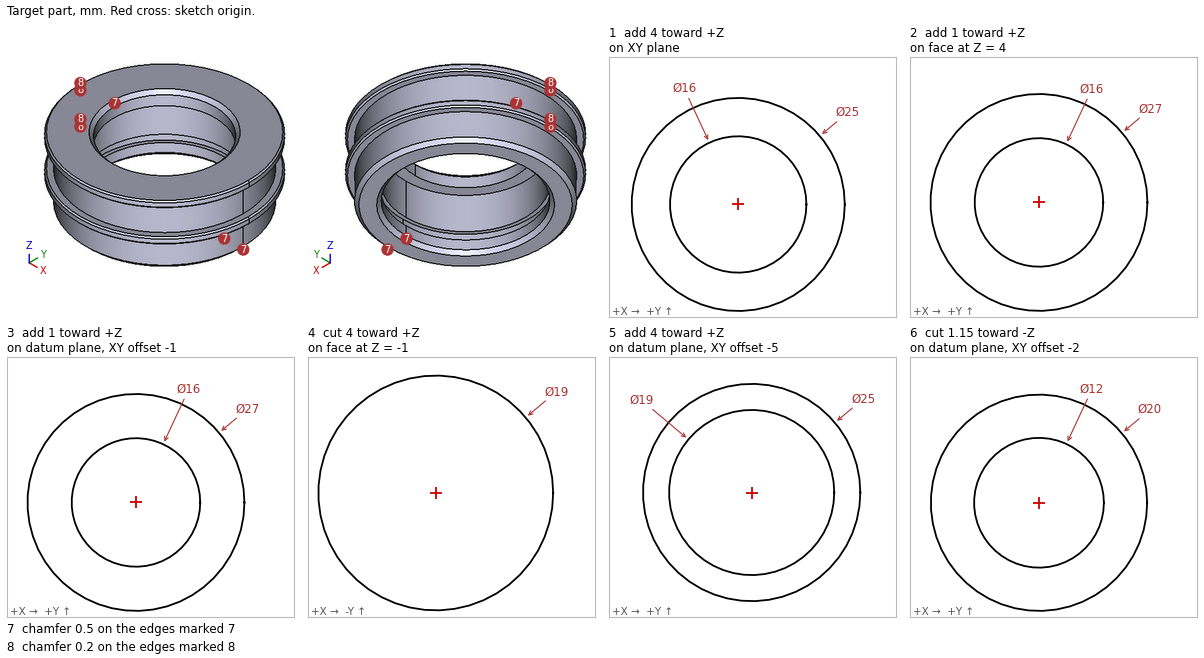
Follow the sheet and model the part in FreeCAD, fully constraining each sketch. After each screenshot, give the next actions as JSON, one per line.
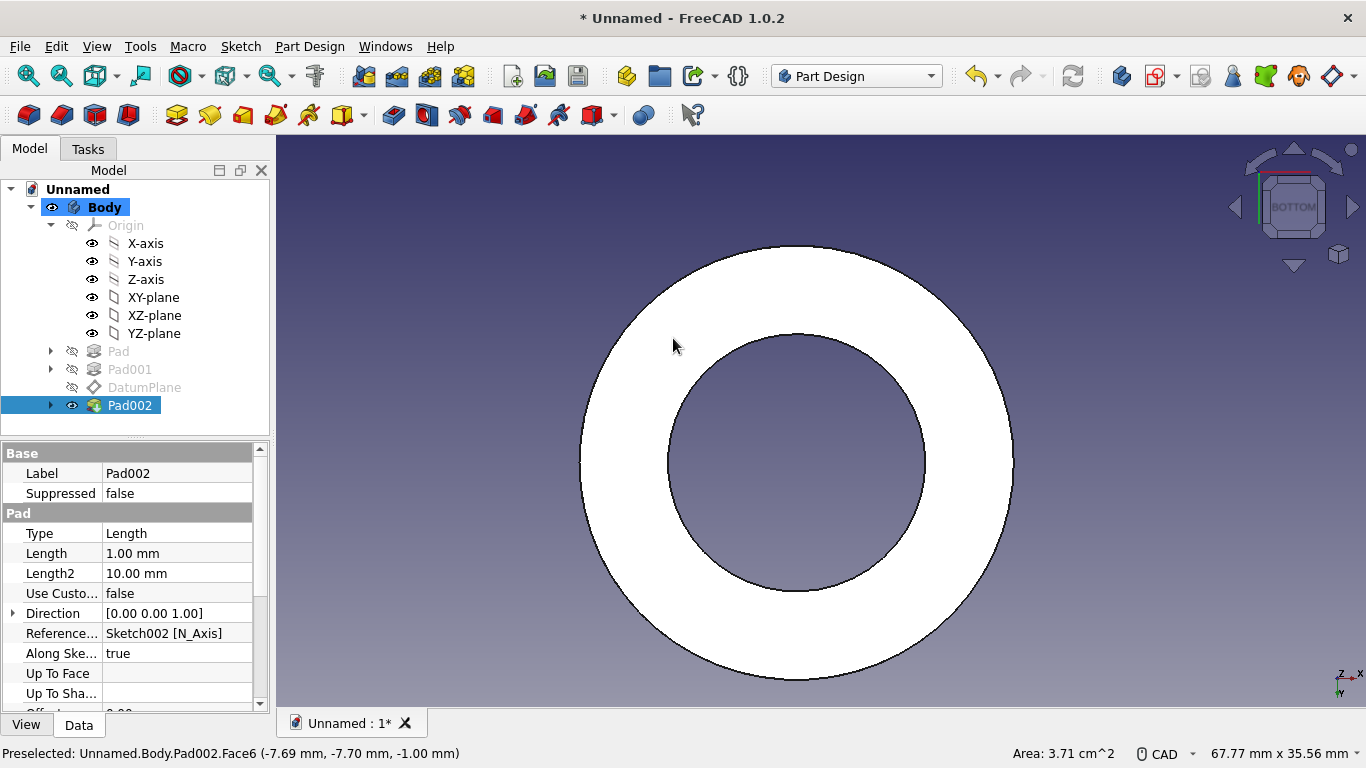
{"action": "left_click", "coordinate": [1154, 76]}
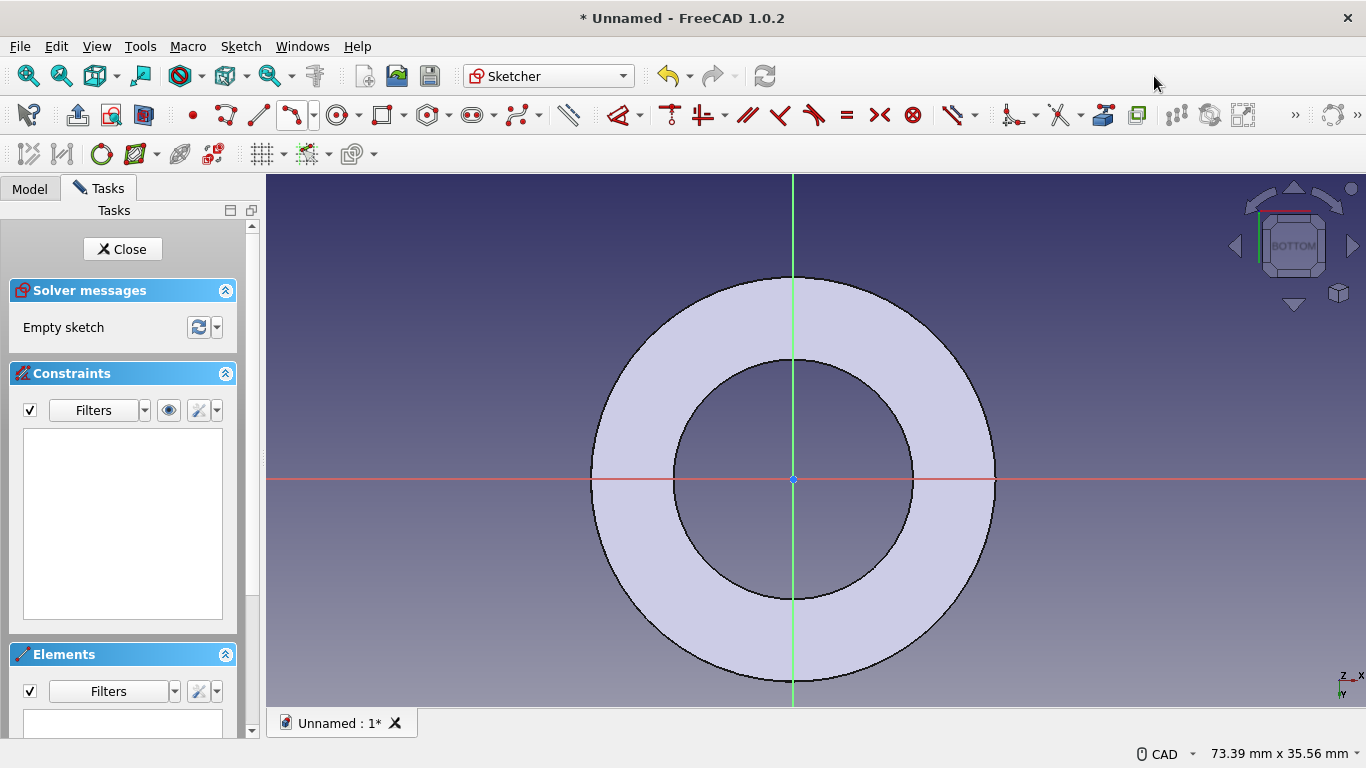
{"action": "left_click", "coordinate": [336, 116]}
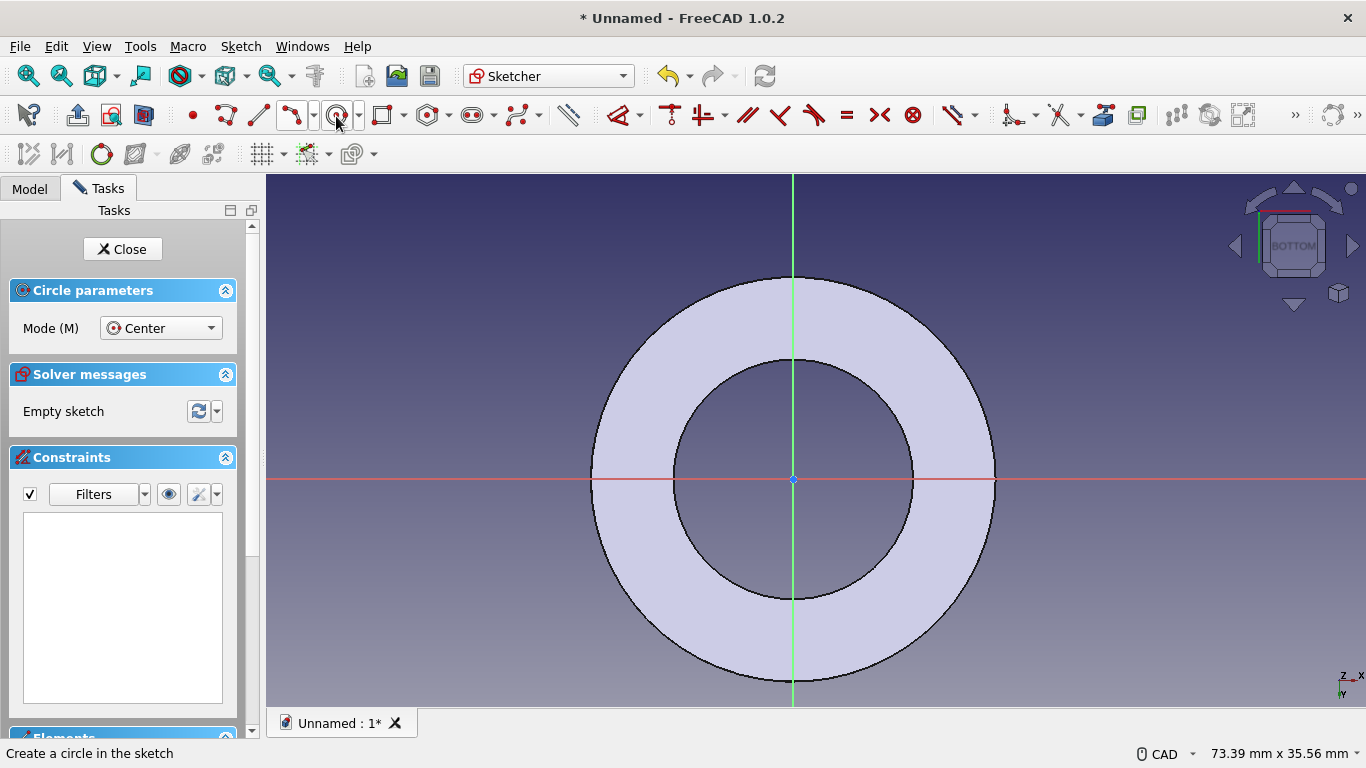
{"action": "left_click", "coordinate": [793, 479]}
{"action": "left_click", "coordinate": [894, 379]}
{"action": "key", "text": "Escape"}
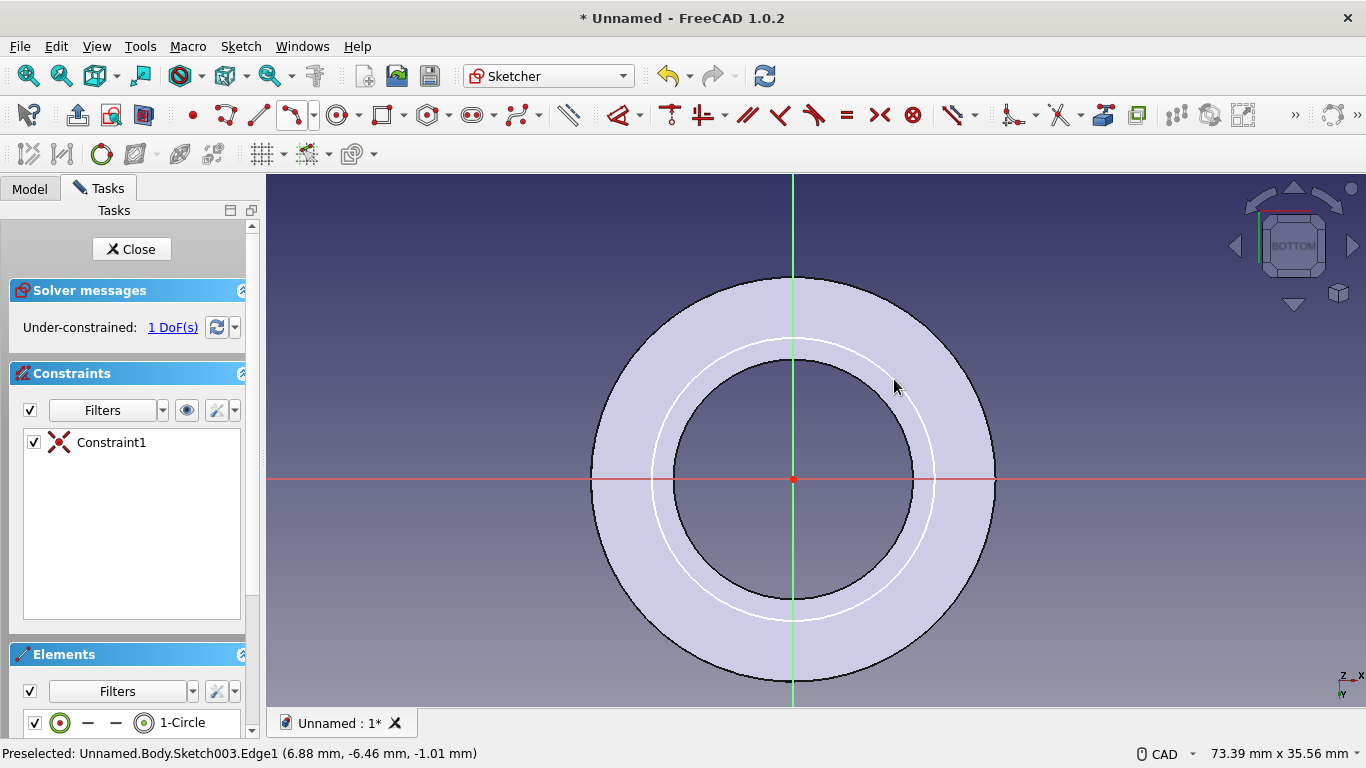
{"action": "left_click", "coordinate": [618, 116]}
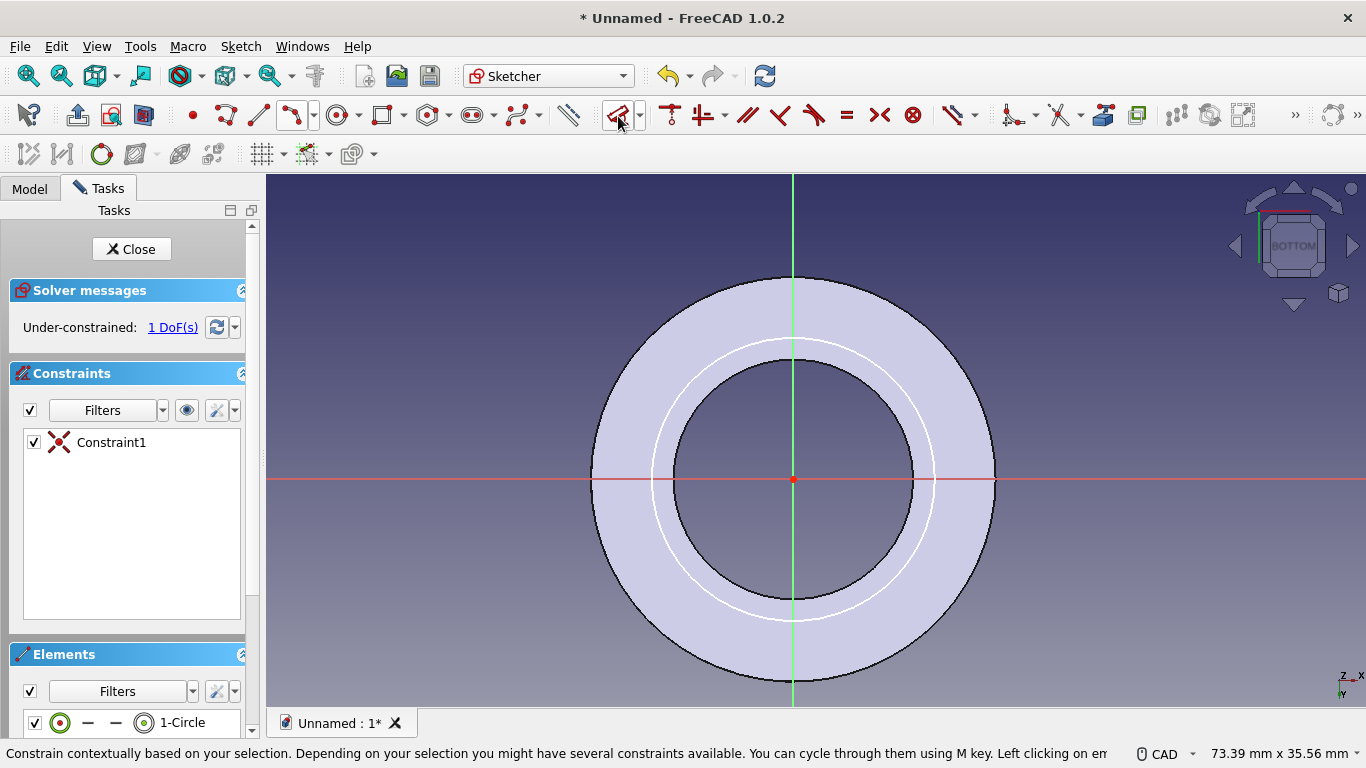
{"action": "left_click", "coordinate": [893, 379]}
{"action": "left_click", "coordinate": [916, 356]}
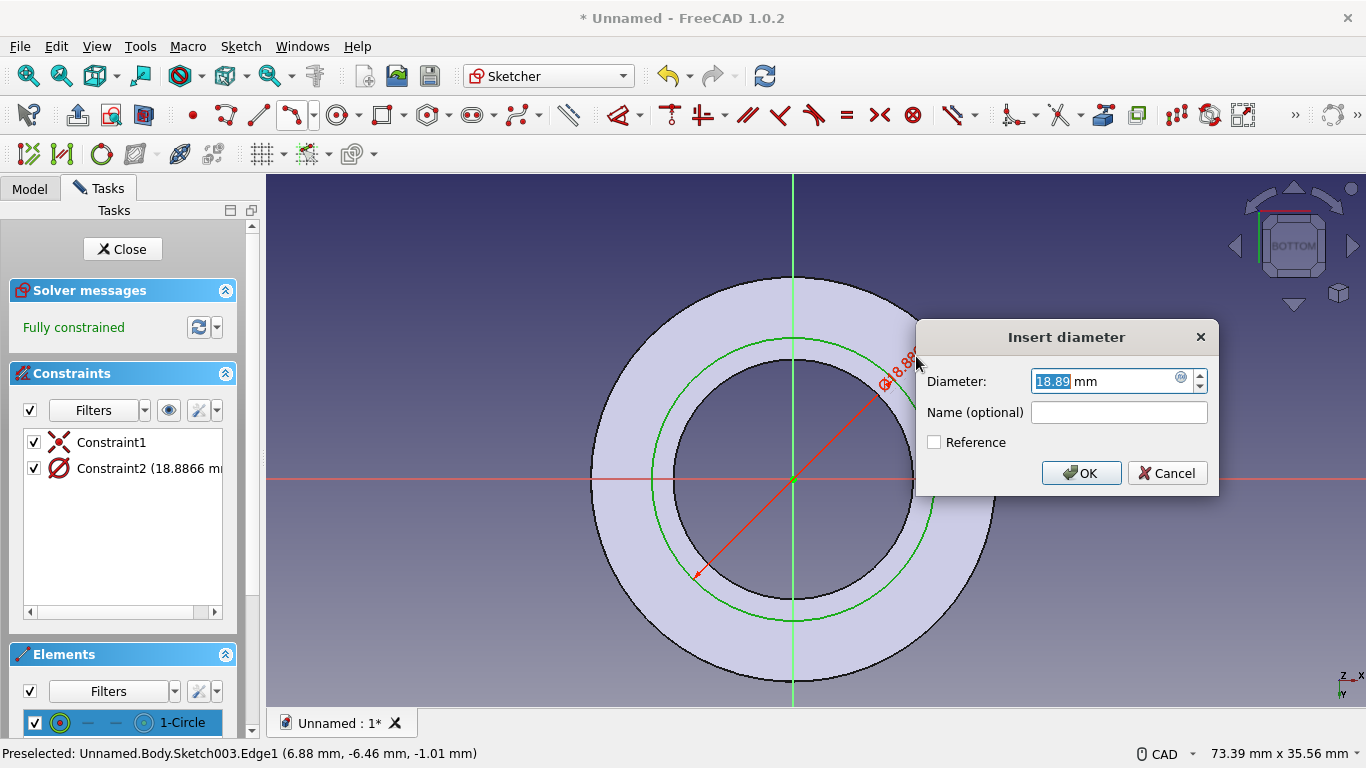
{"action": "type", "text": "19"}
{"action": "key", "text": "Return"}
{"action": "key", "text": "Escape"}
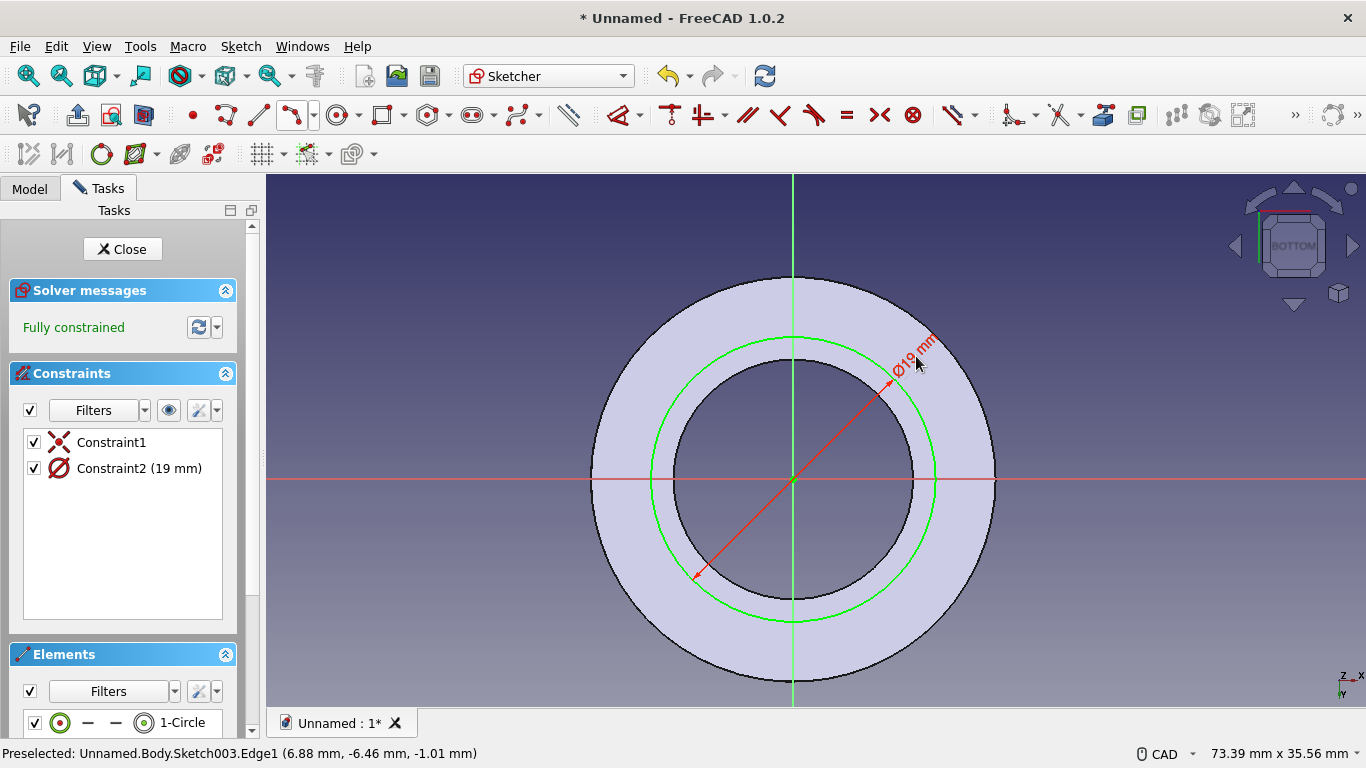
{"action": "left_click", "coordinate": [123, 249]}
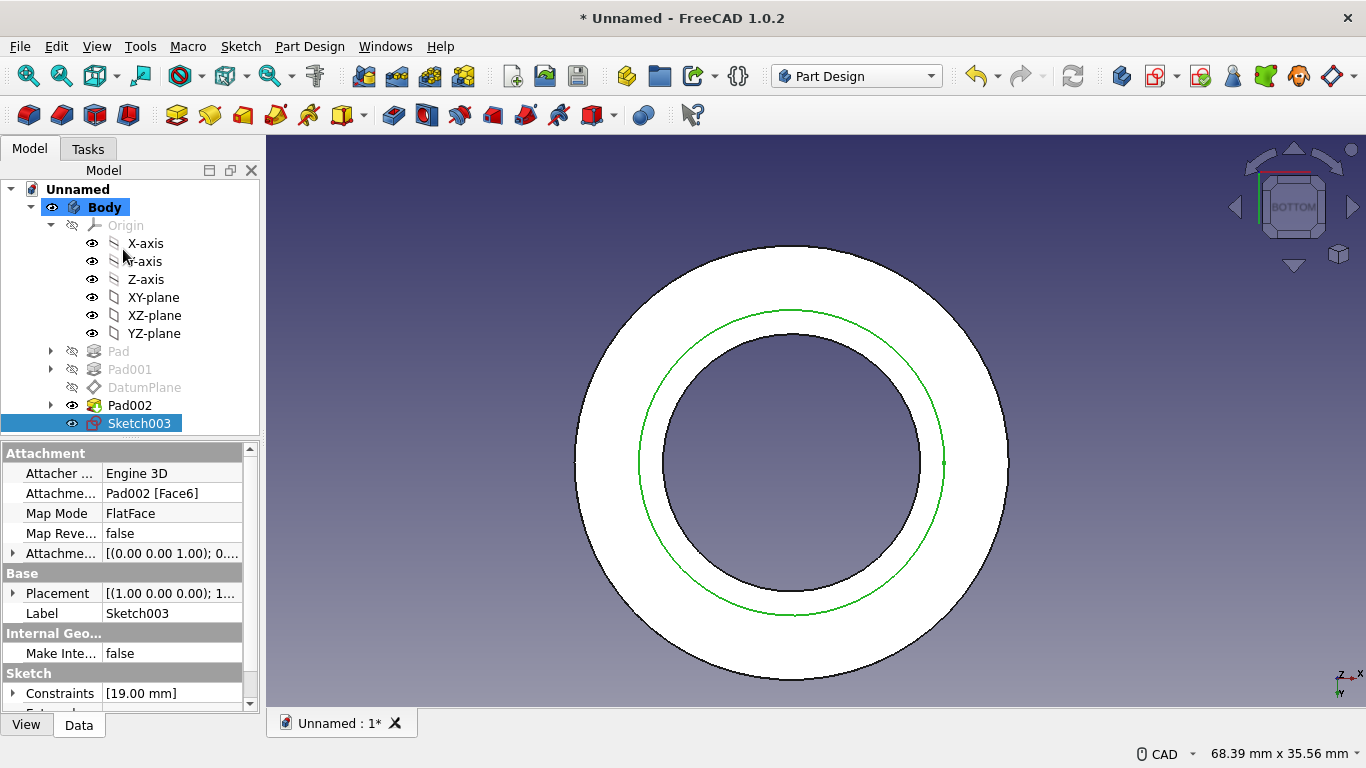
{"action": "left_click", "coordinate": [394, 116]}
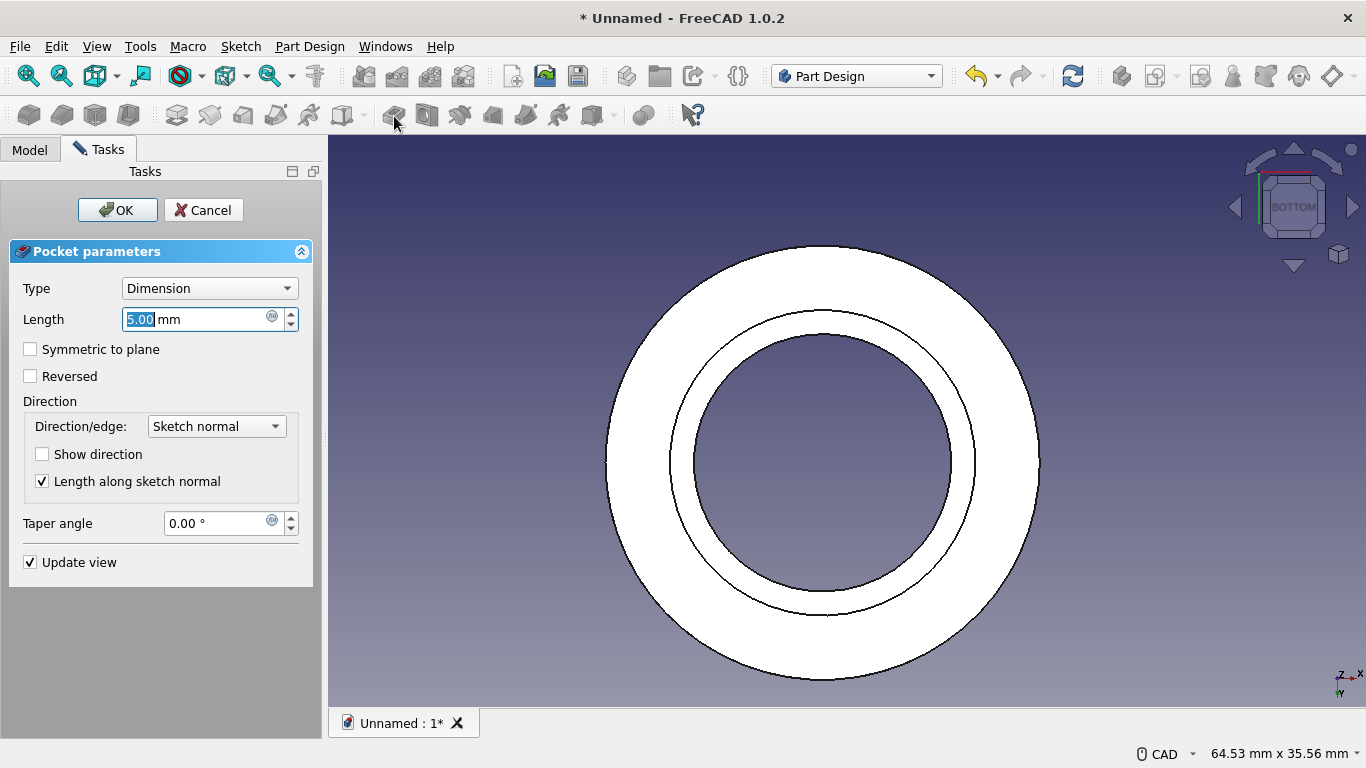
{"action": "type", "text": "4"}
{"action": "key", "text": "Tab"}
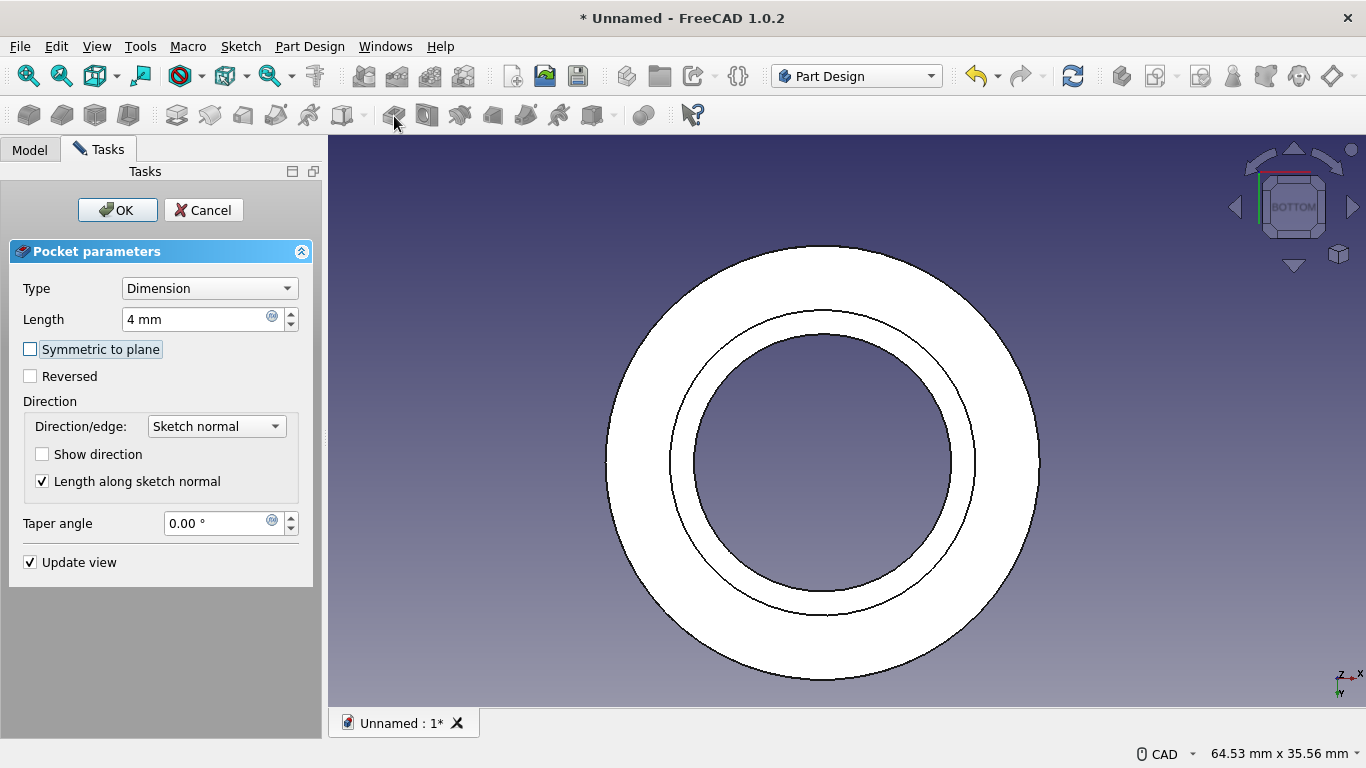
{"action": "left_click", "coordinate": [118, 210]}